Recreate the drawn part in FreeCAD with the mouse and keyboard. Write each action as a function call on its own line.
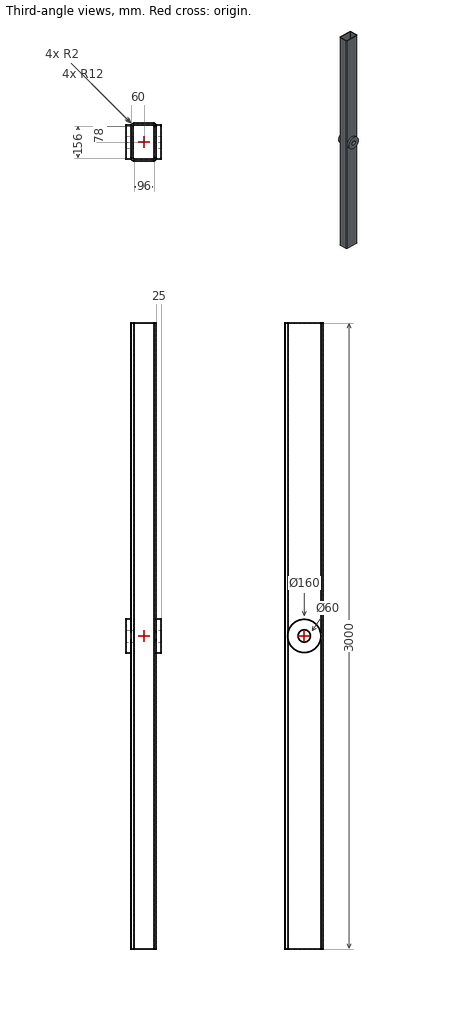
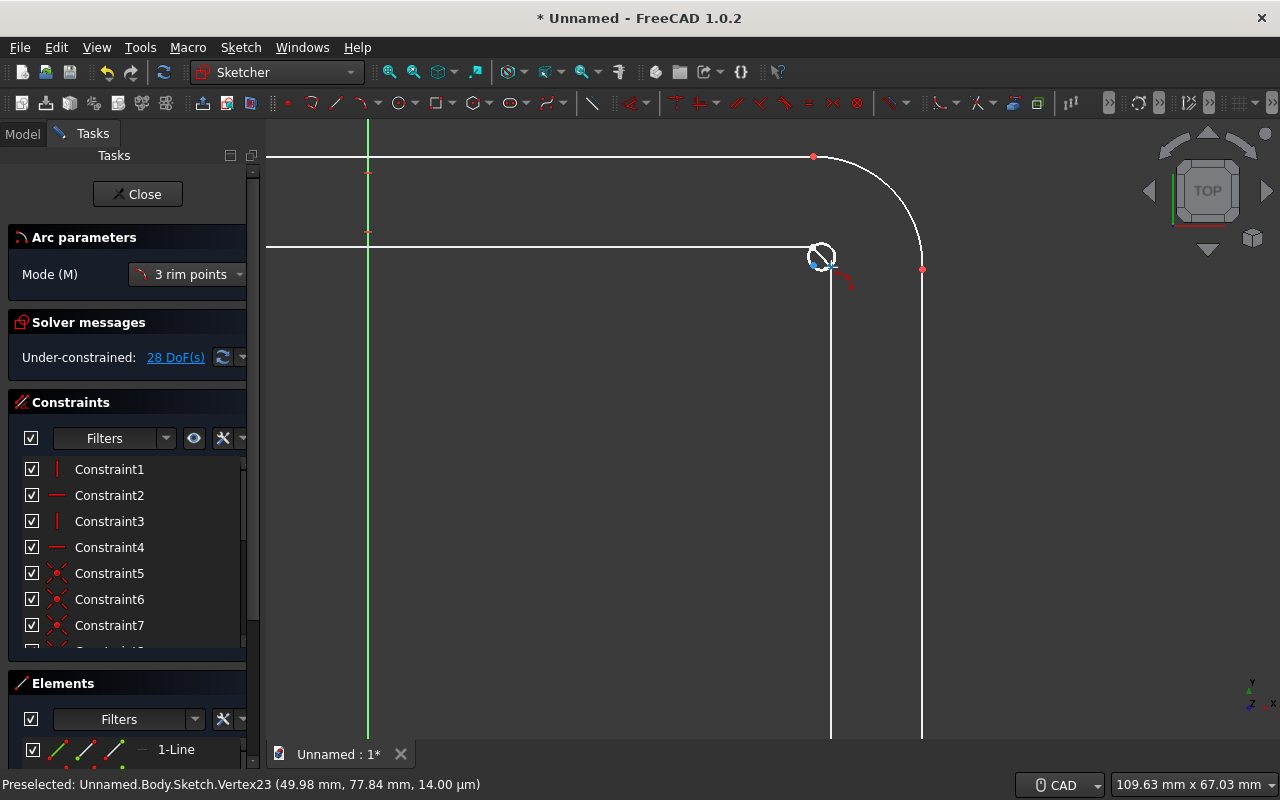
scroll(825, 252, up, 6)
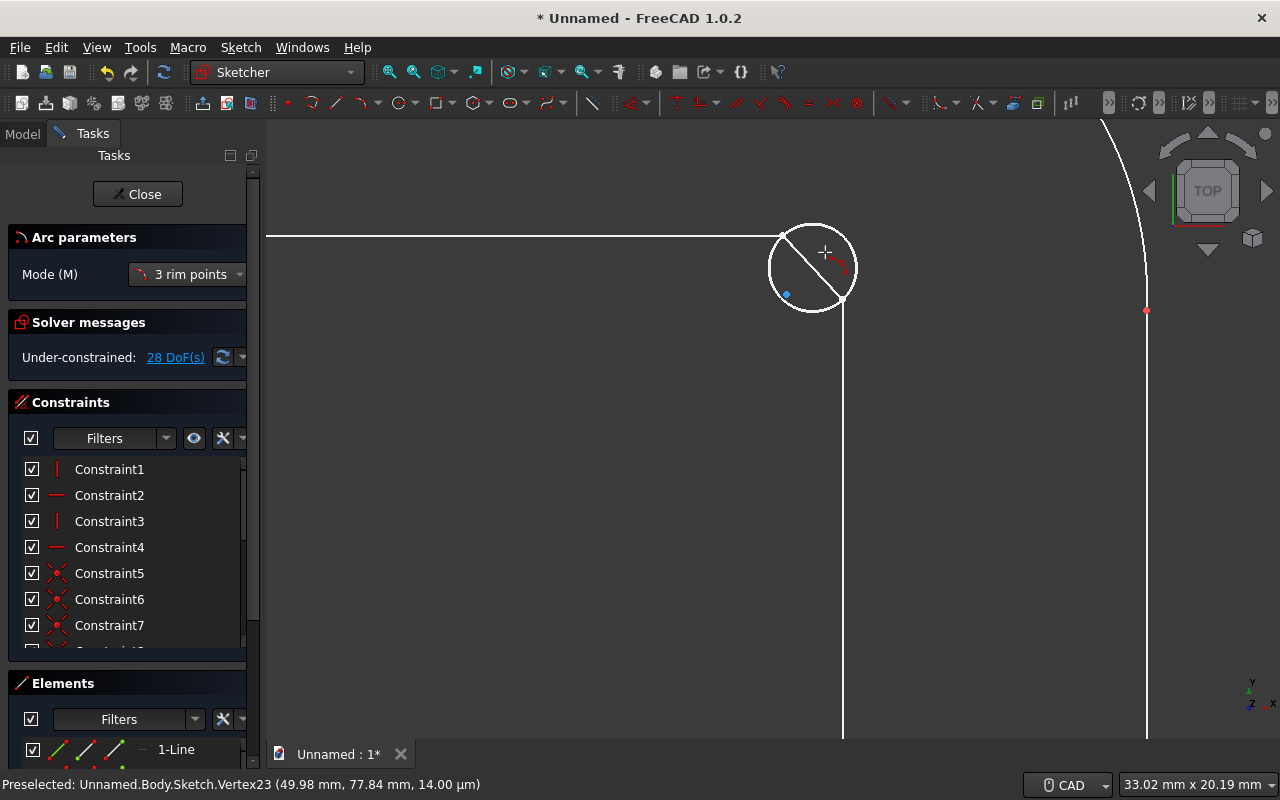
click(825, 252)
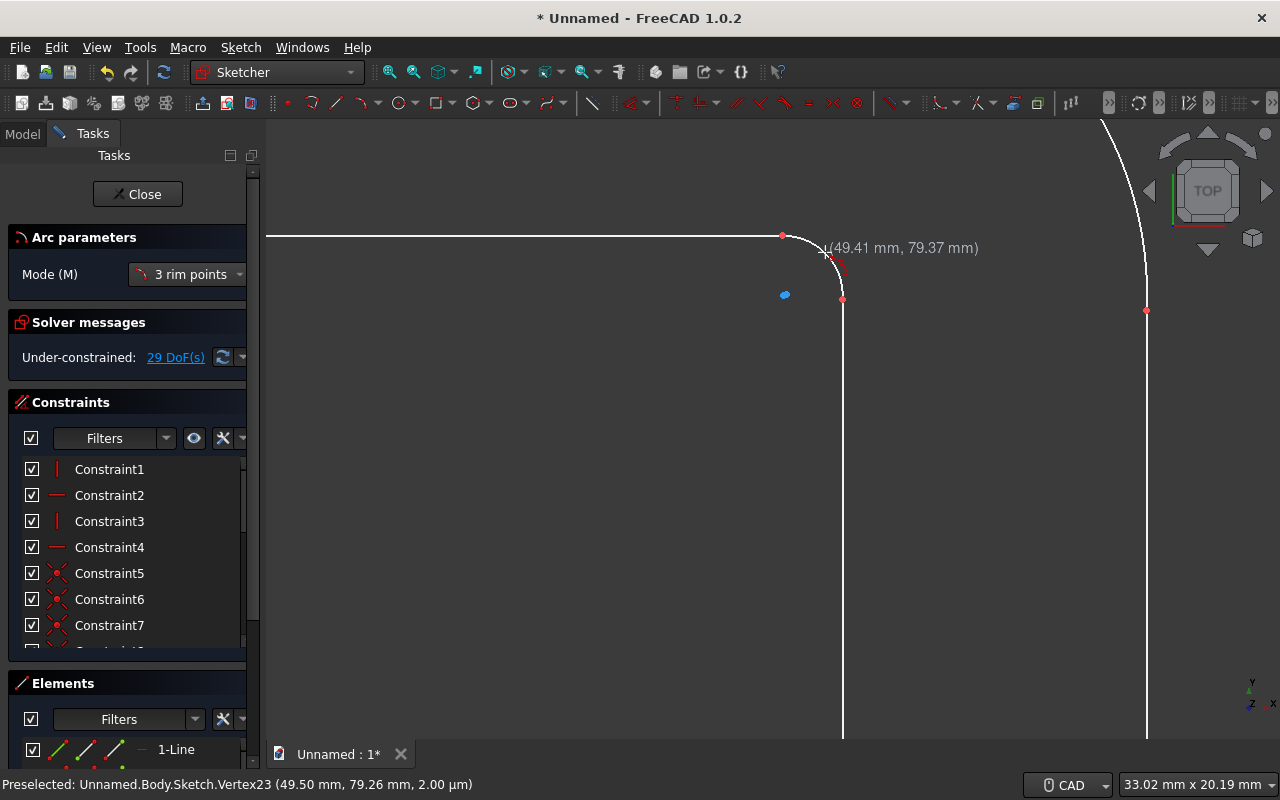
scroll(817, 248, down, 13)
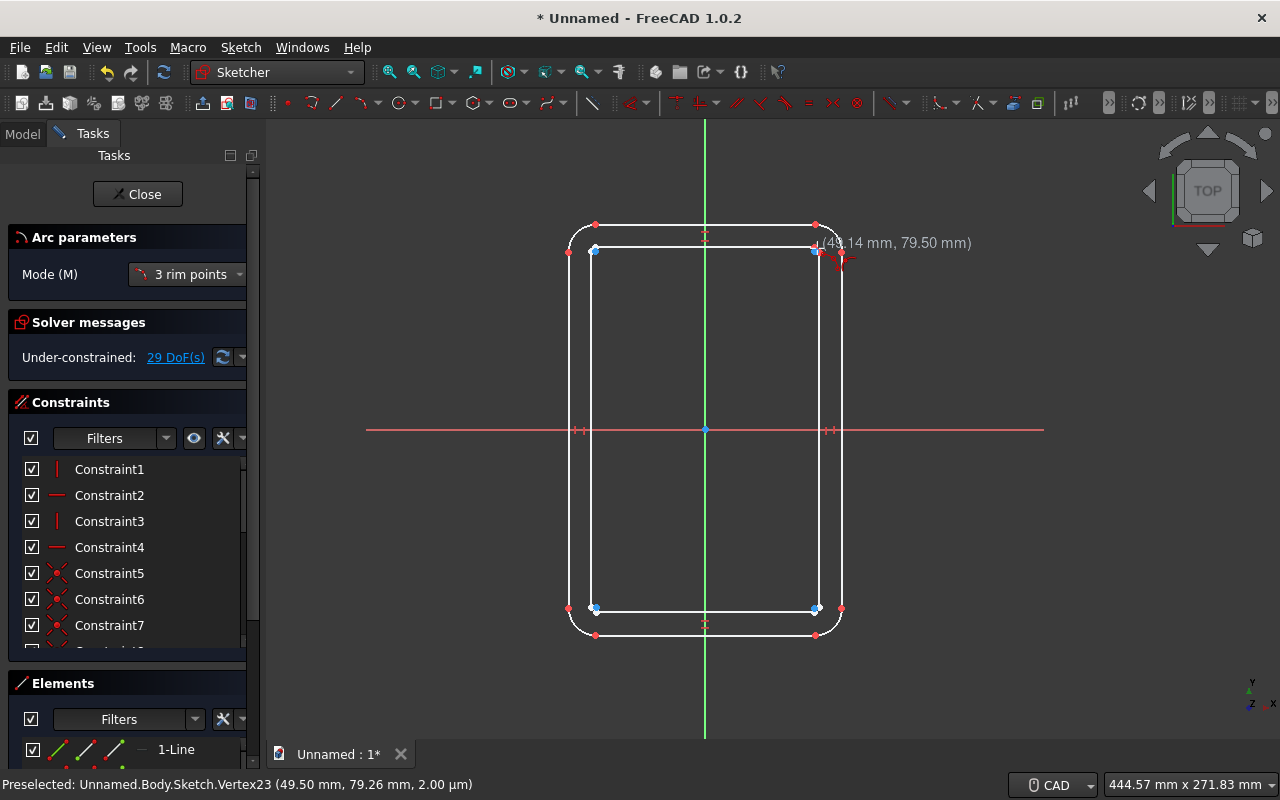
scroll(819, 607, up, 7)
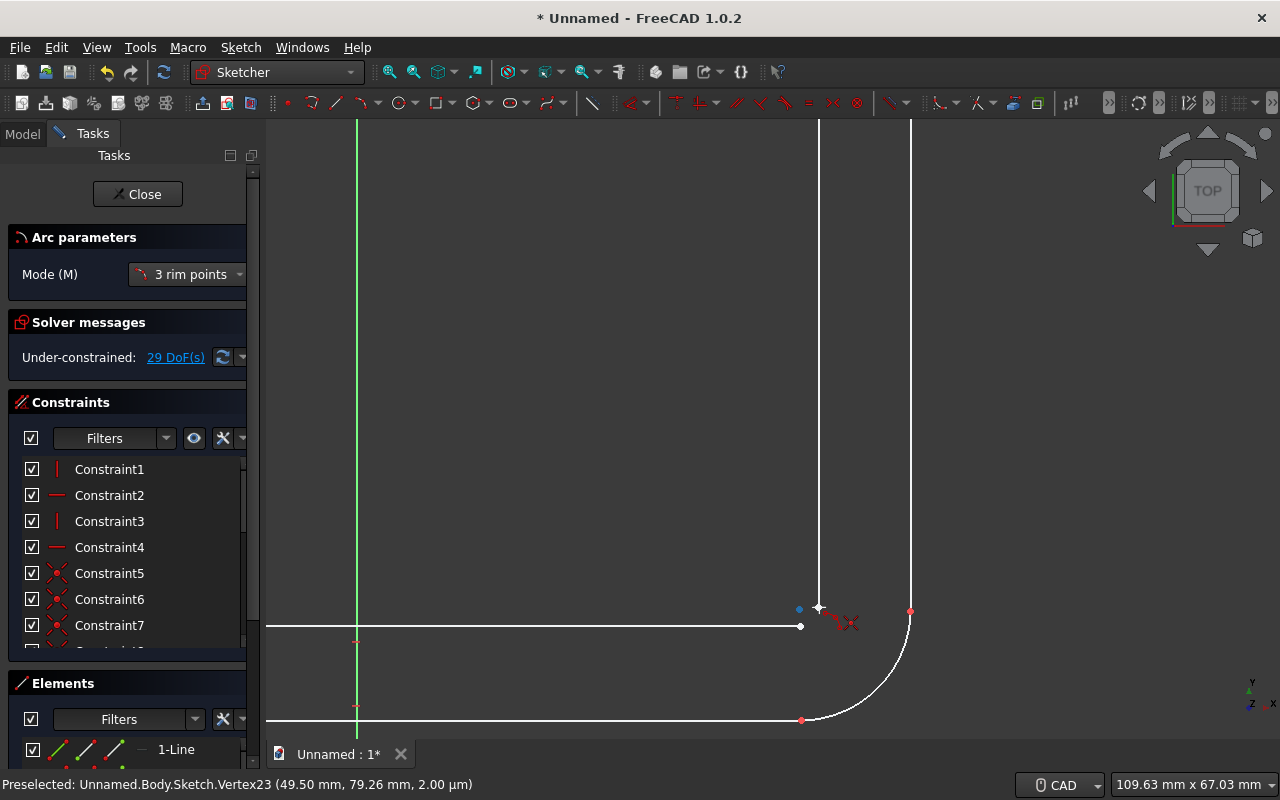
click(819, 607)
click(800, 626)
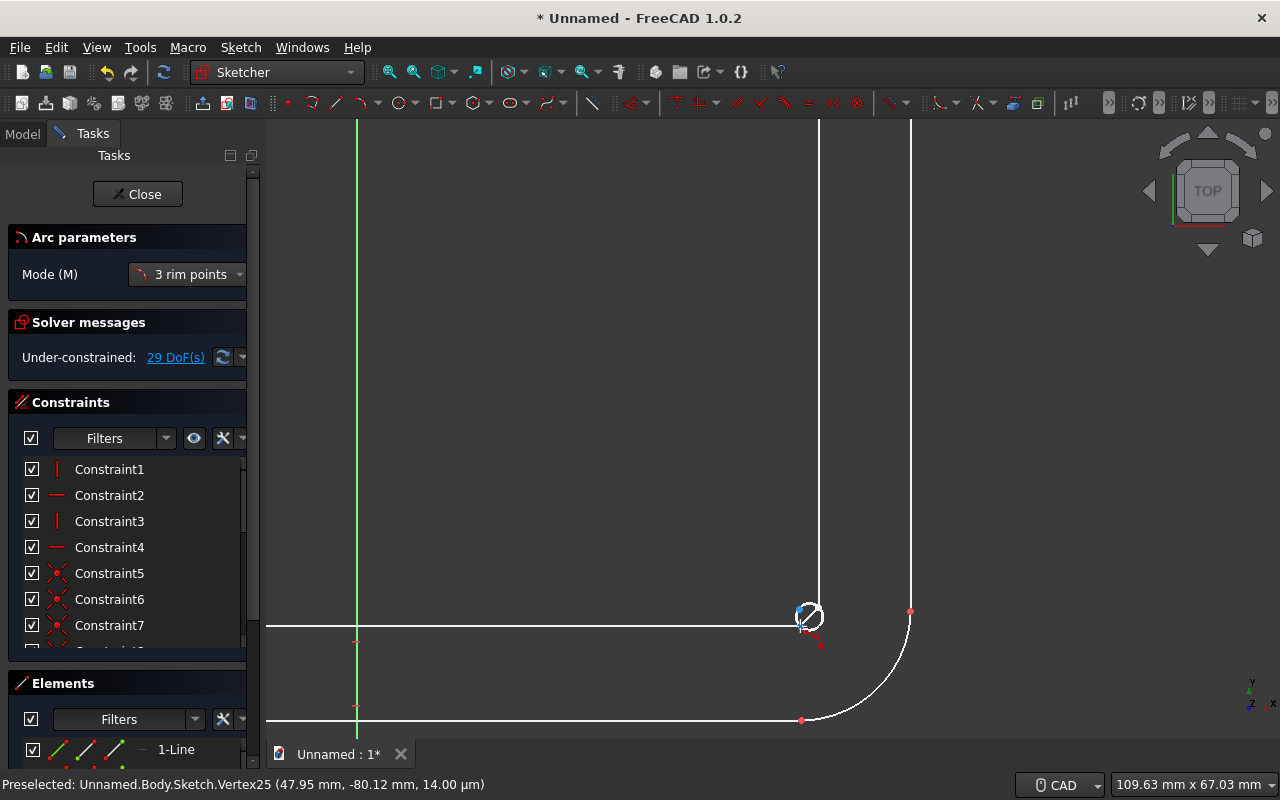
scroll(814, 620, up, 6)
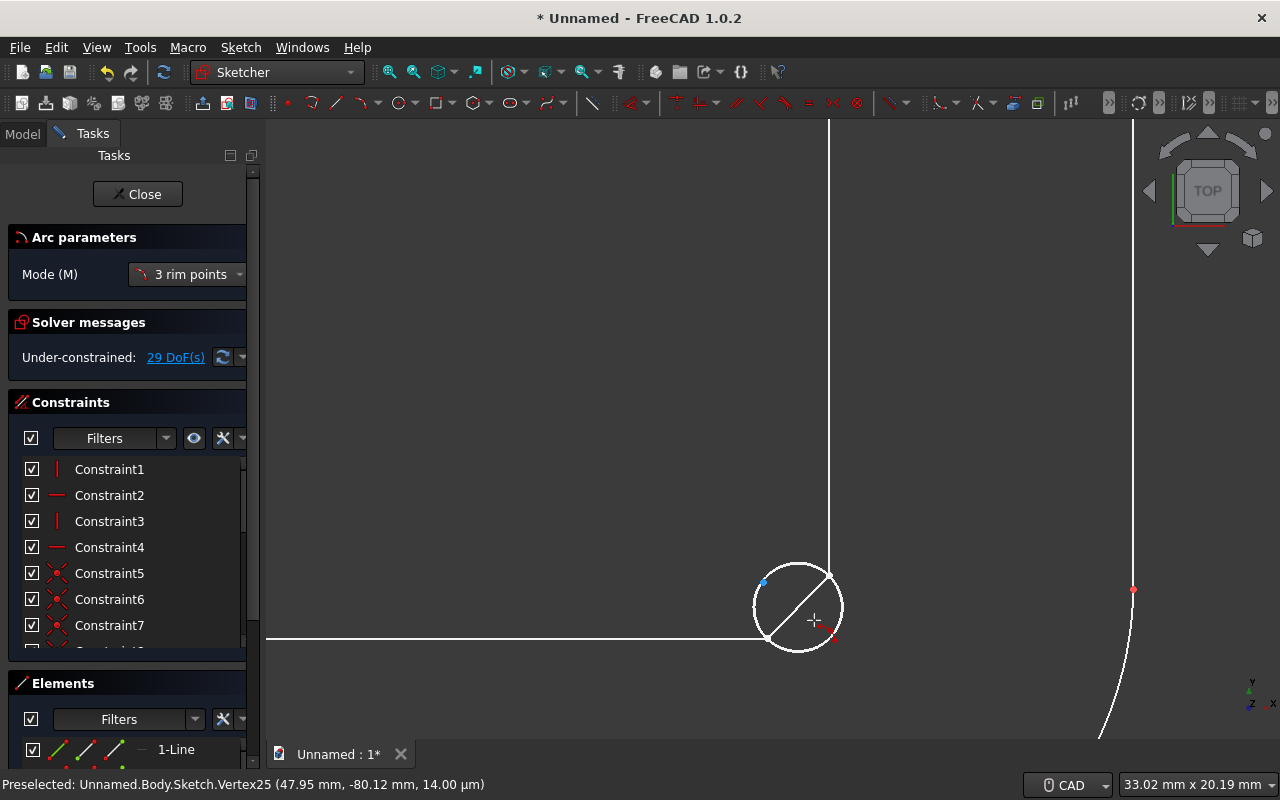
click(812, 617)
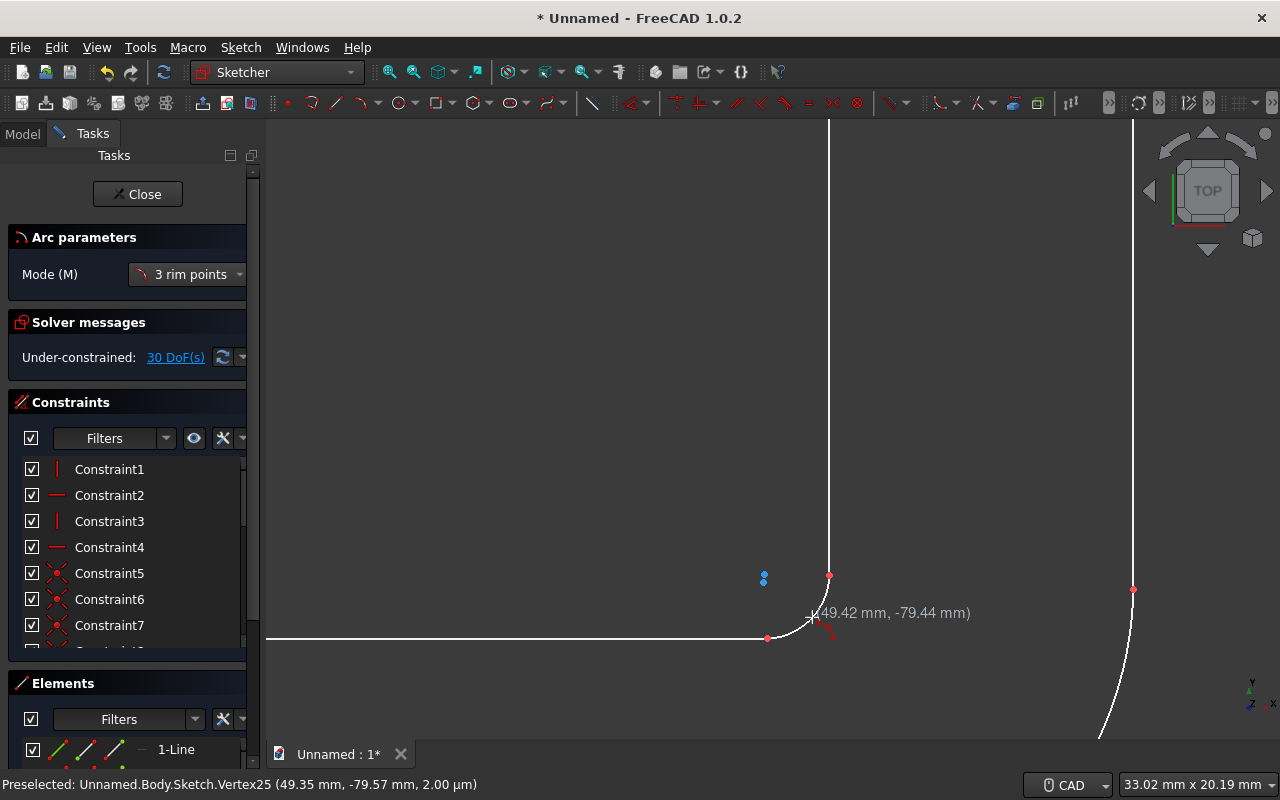
scroll(818, 610, down, 13)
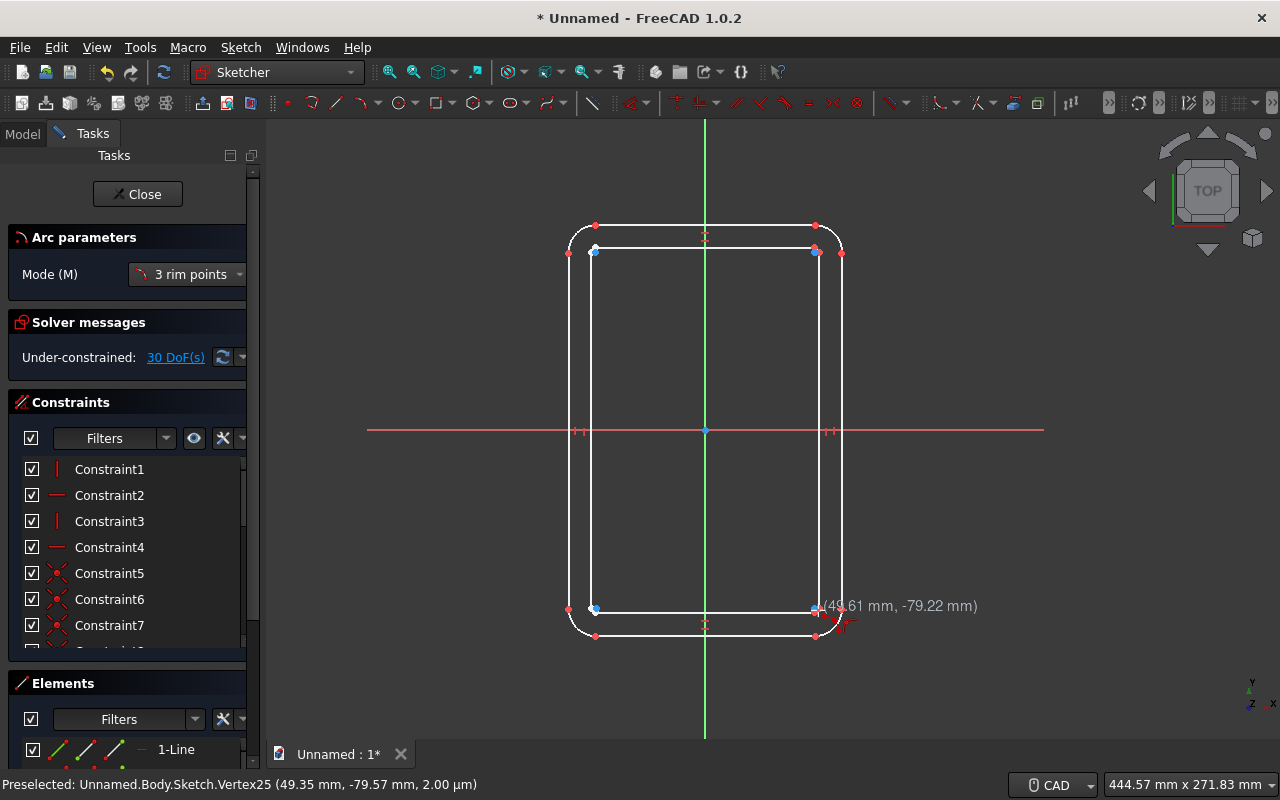
scroll(596, 613, up, 7)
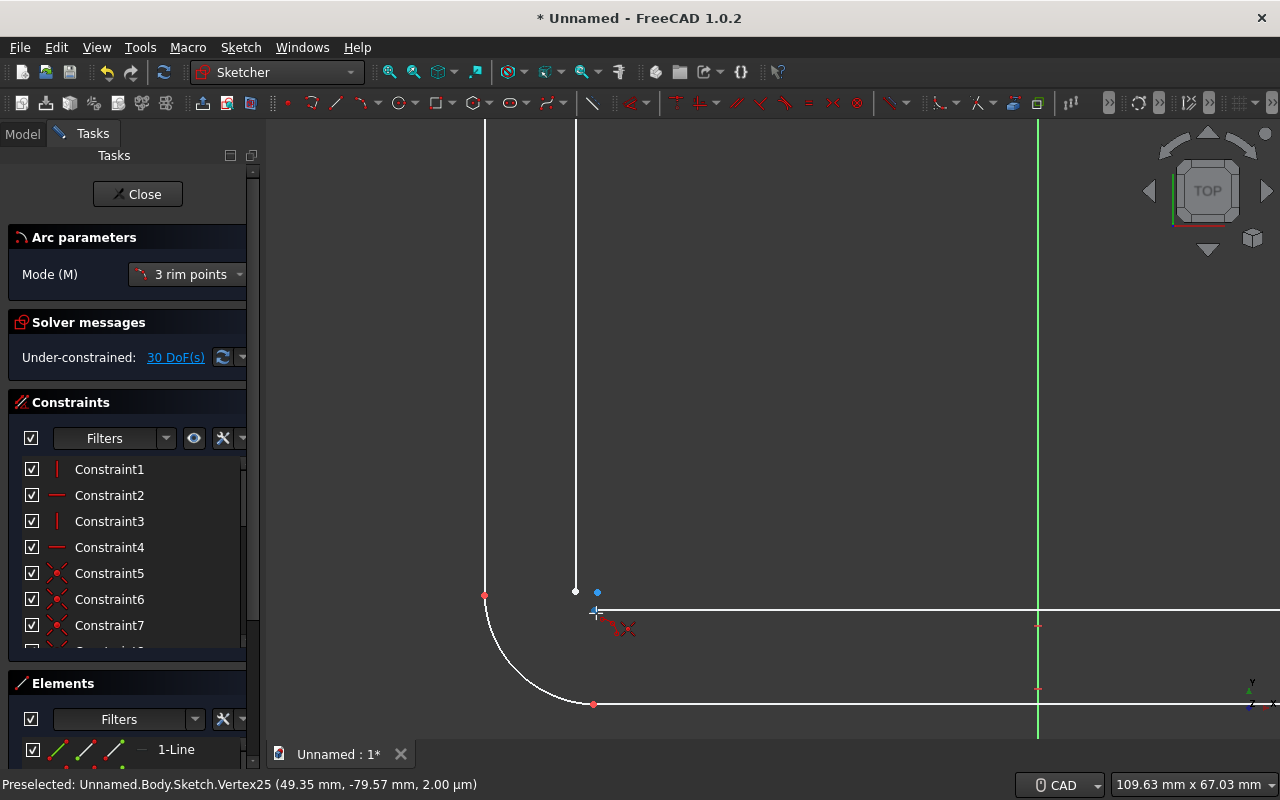
click(595, 610)
click(576, 591)